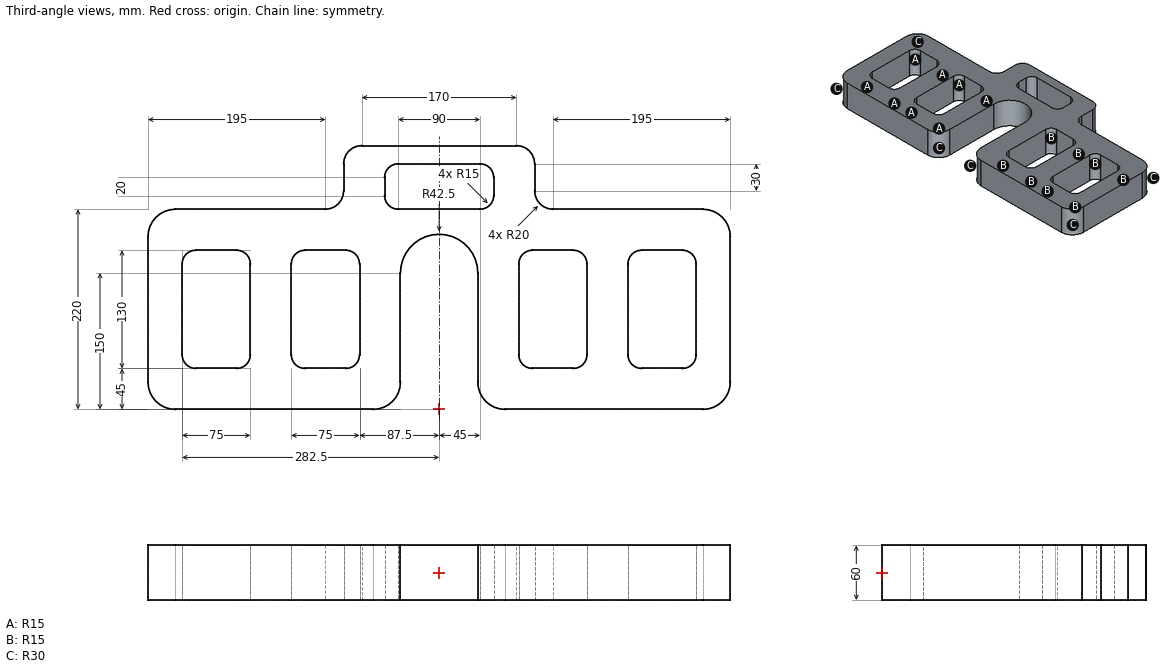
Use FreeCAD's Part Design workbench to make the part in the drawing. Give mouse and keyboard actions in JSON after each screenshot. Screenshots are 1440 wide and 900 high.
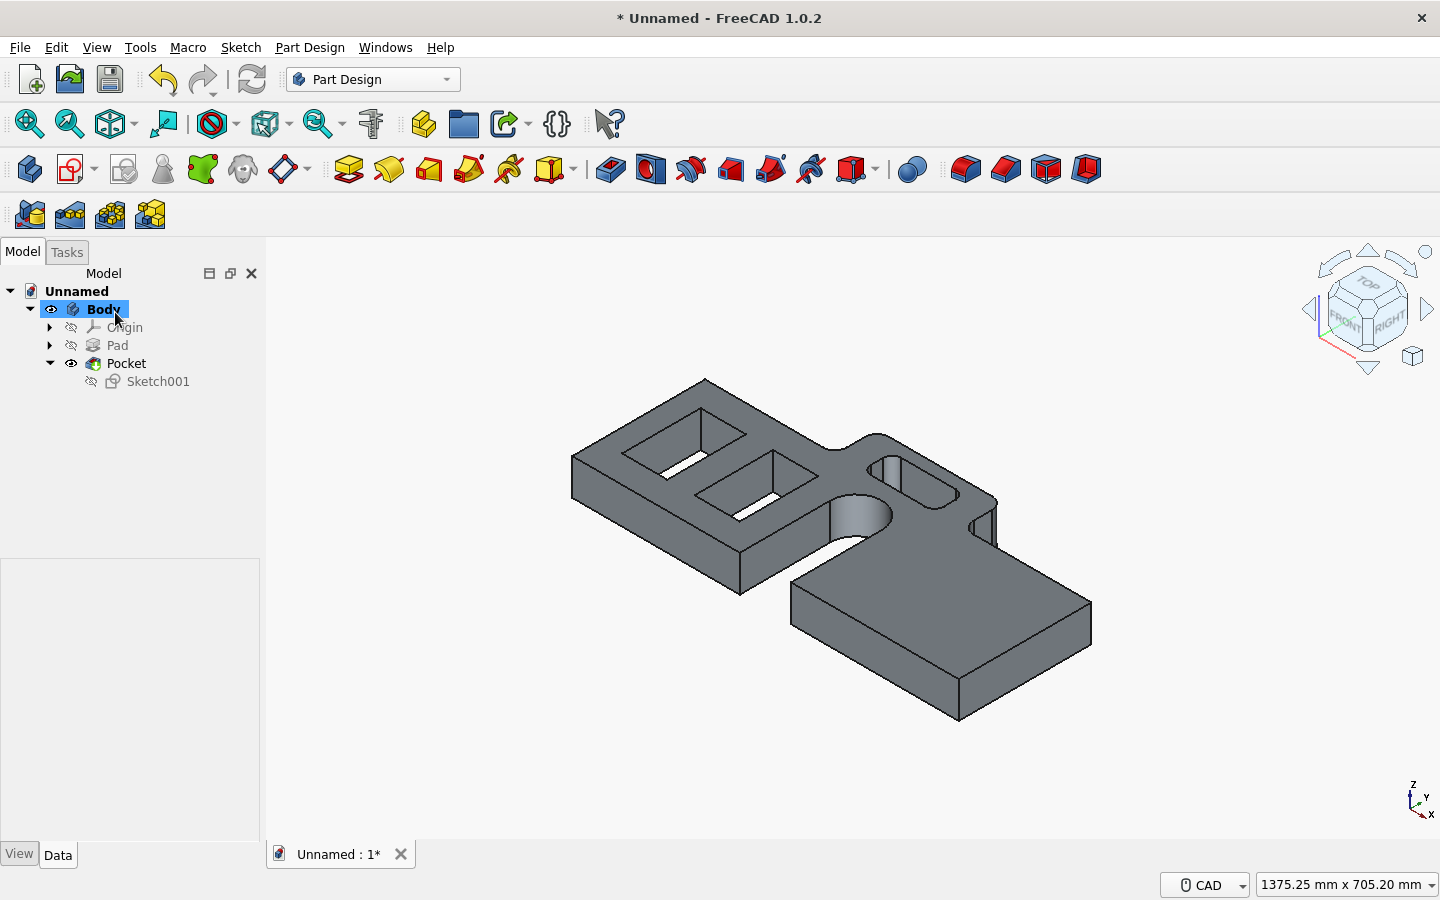
{"action": "key", "text": "2"}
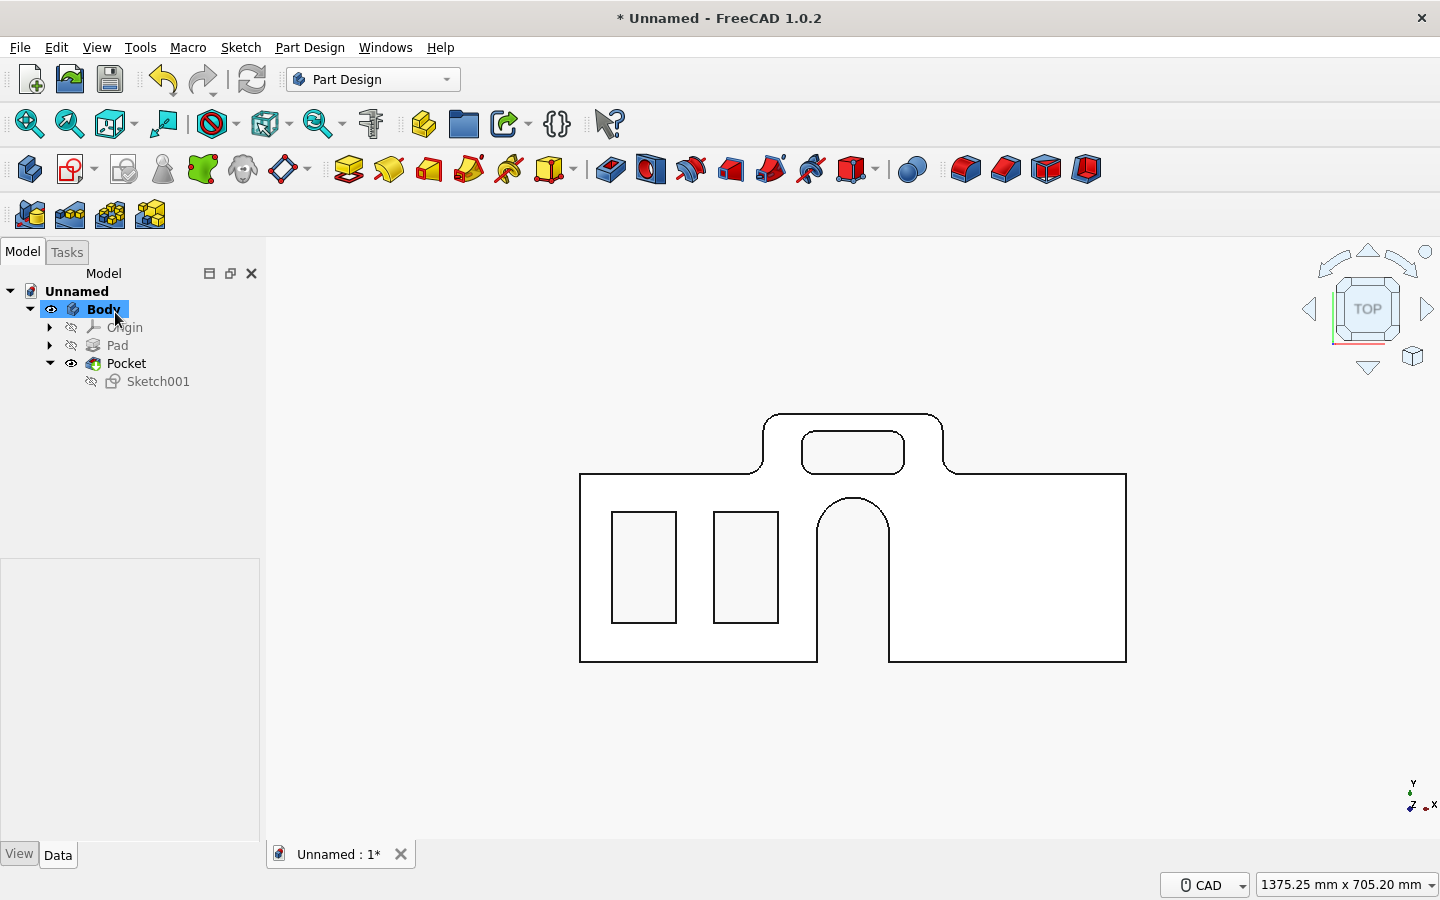
{"action": "key", "text": "1"}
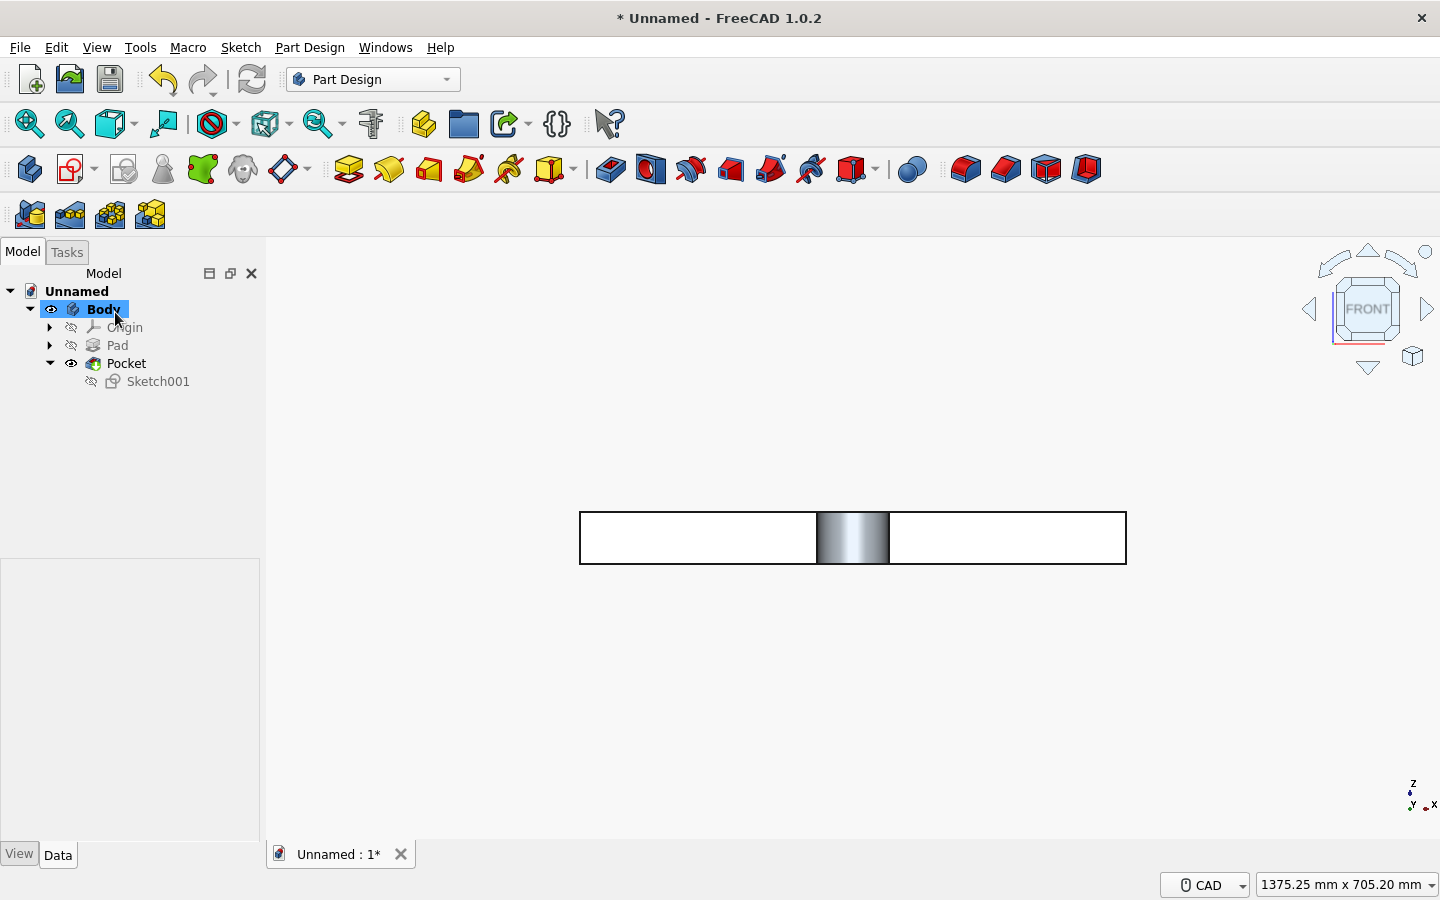
{"action": "key", "text": "3"}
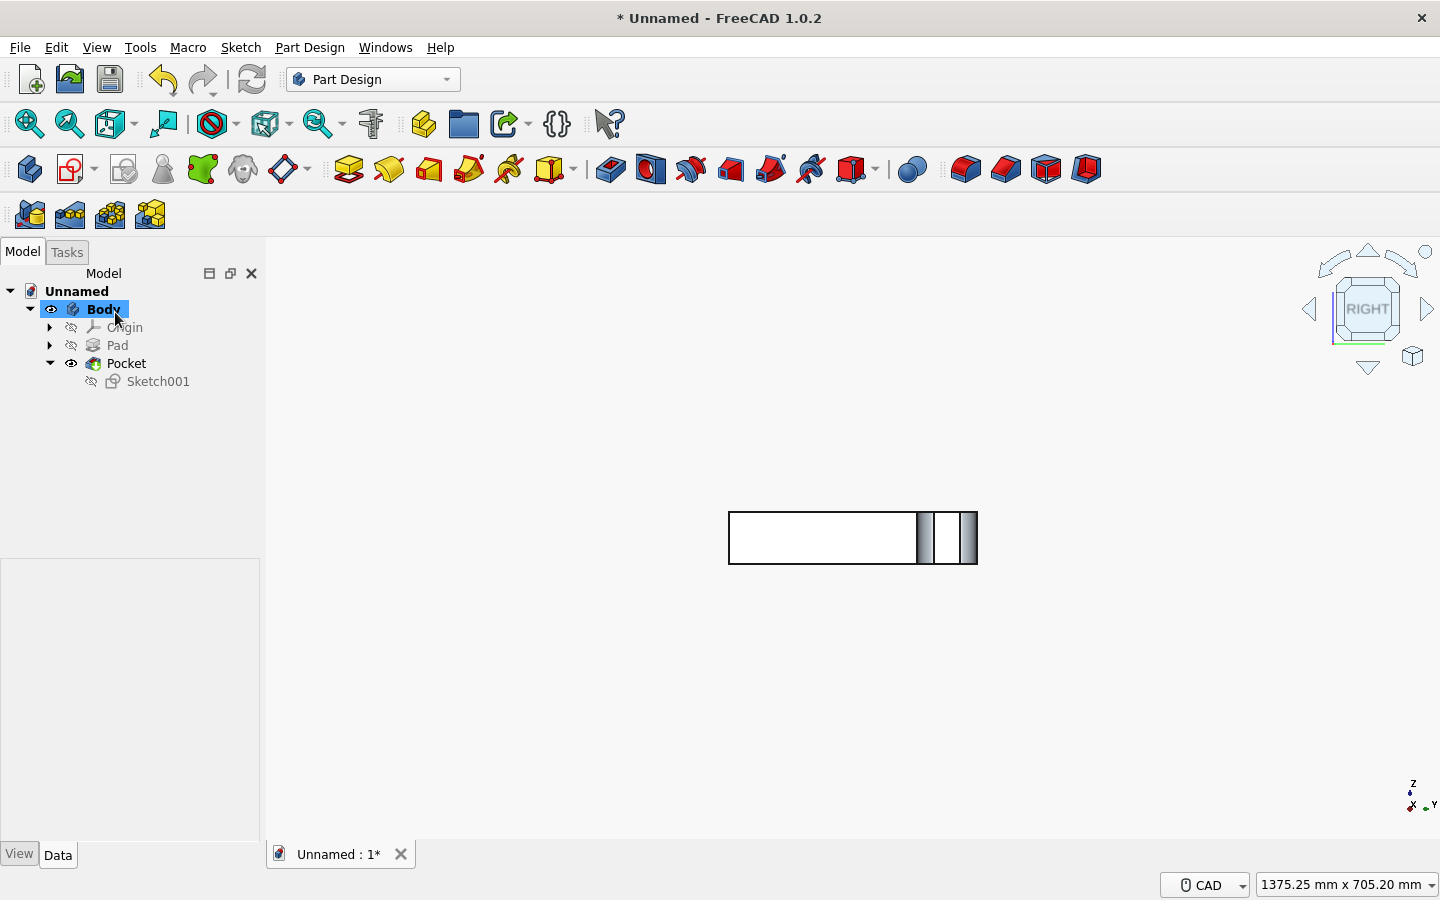
{"action": "key", "text": "v f"}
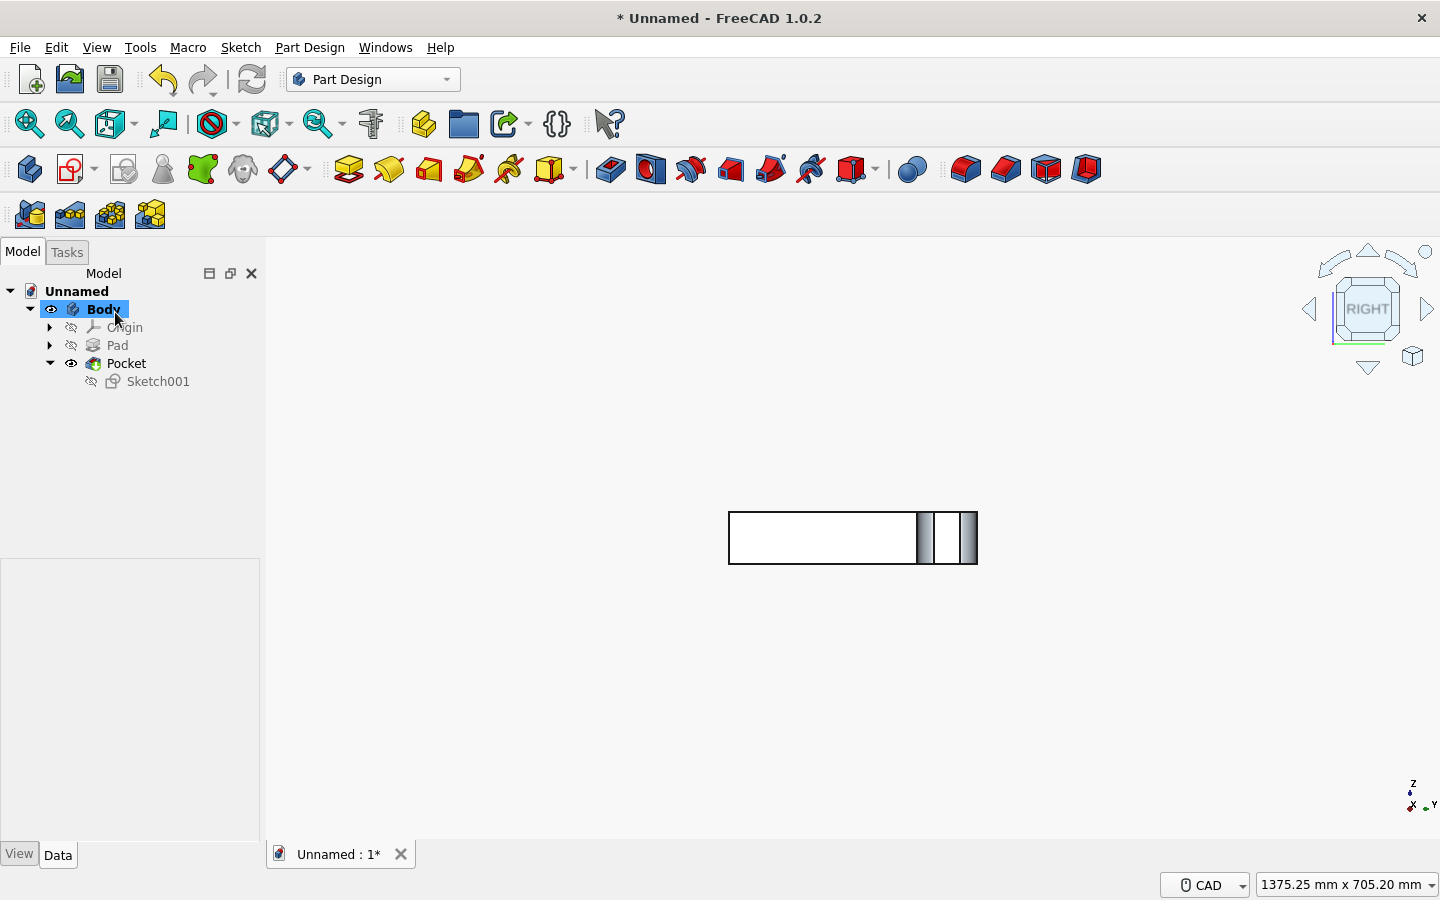
{"action": "key", "text": "5"}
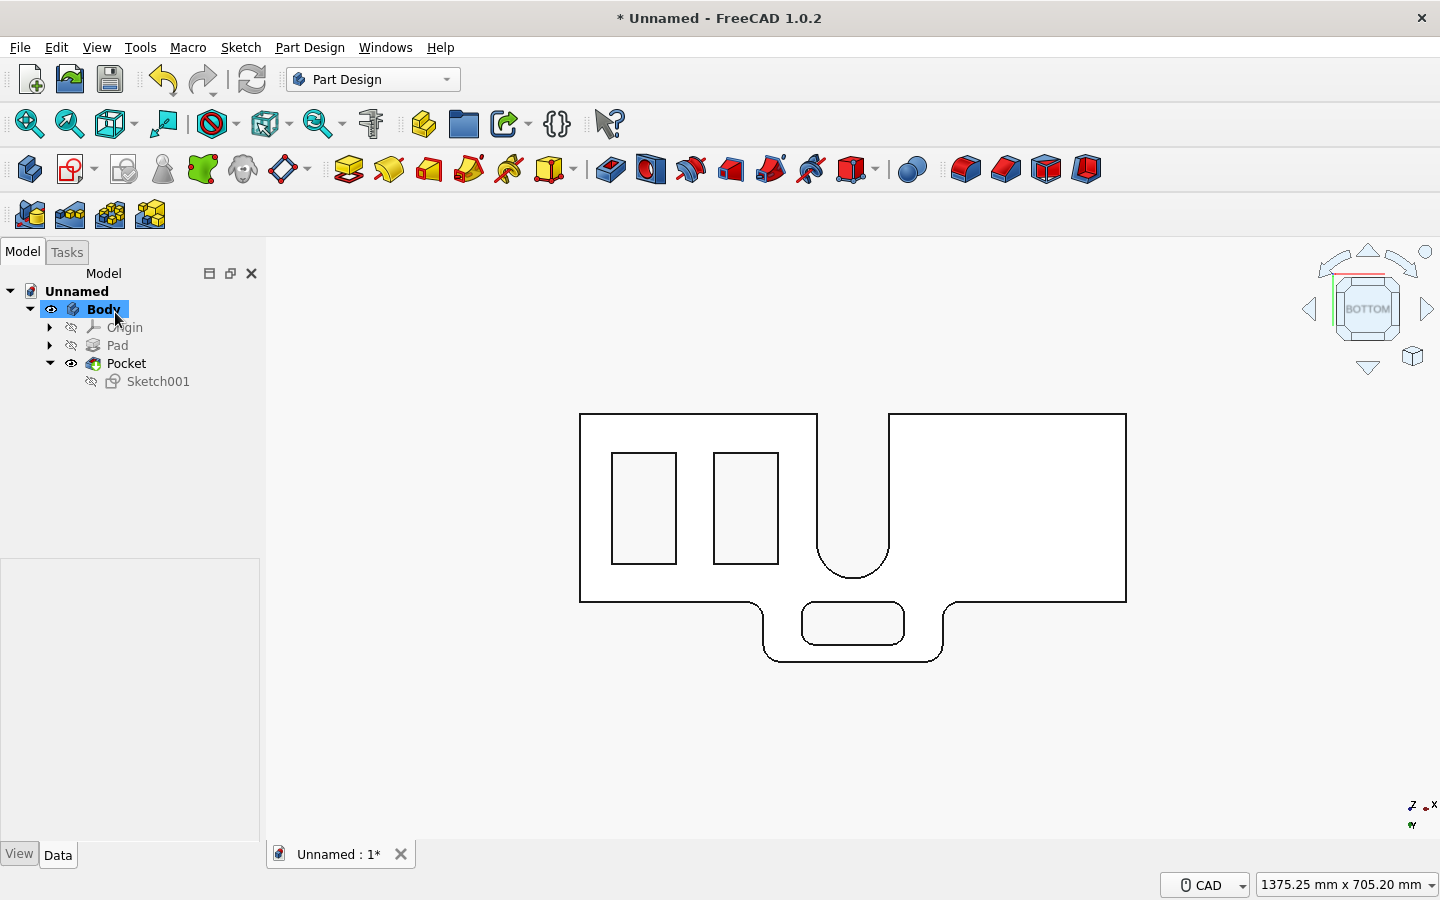
{"action": "key", "text": "4"}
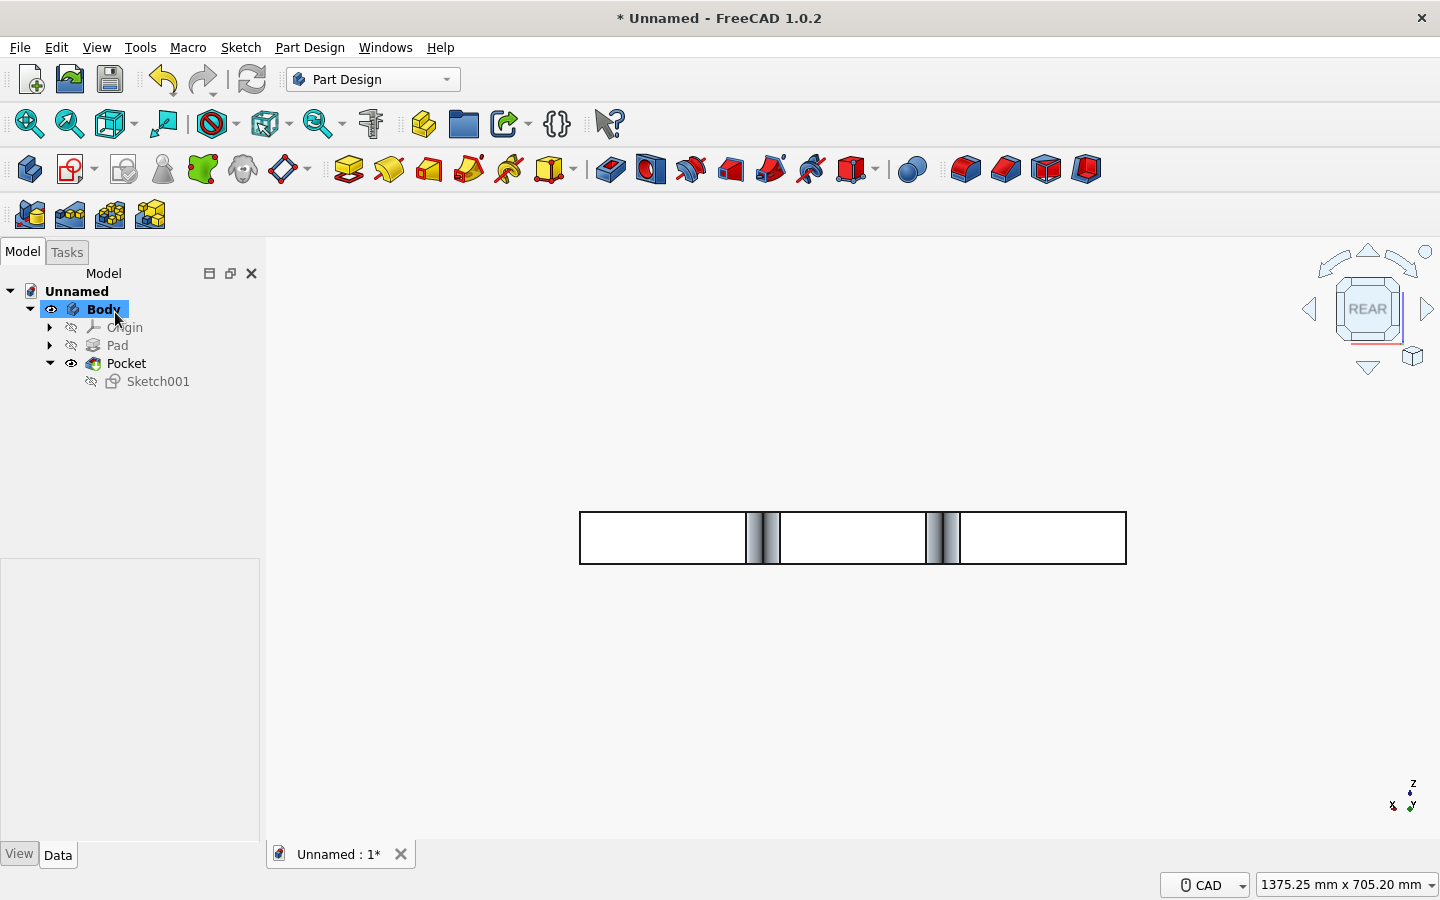
{"action": "key", "text": "6"}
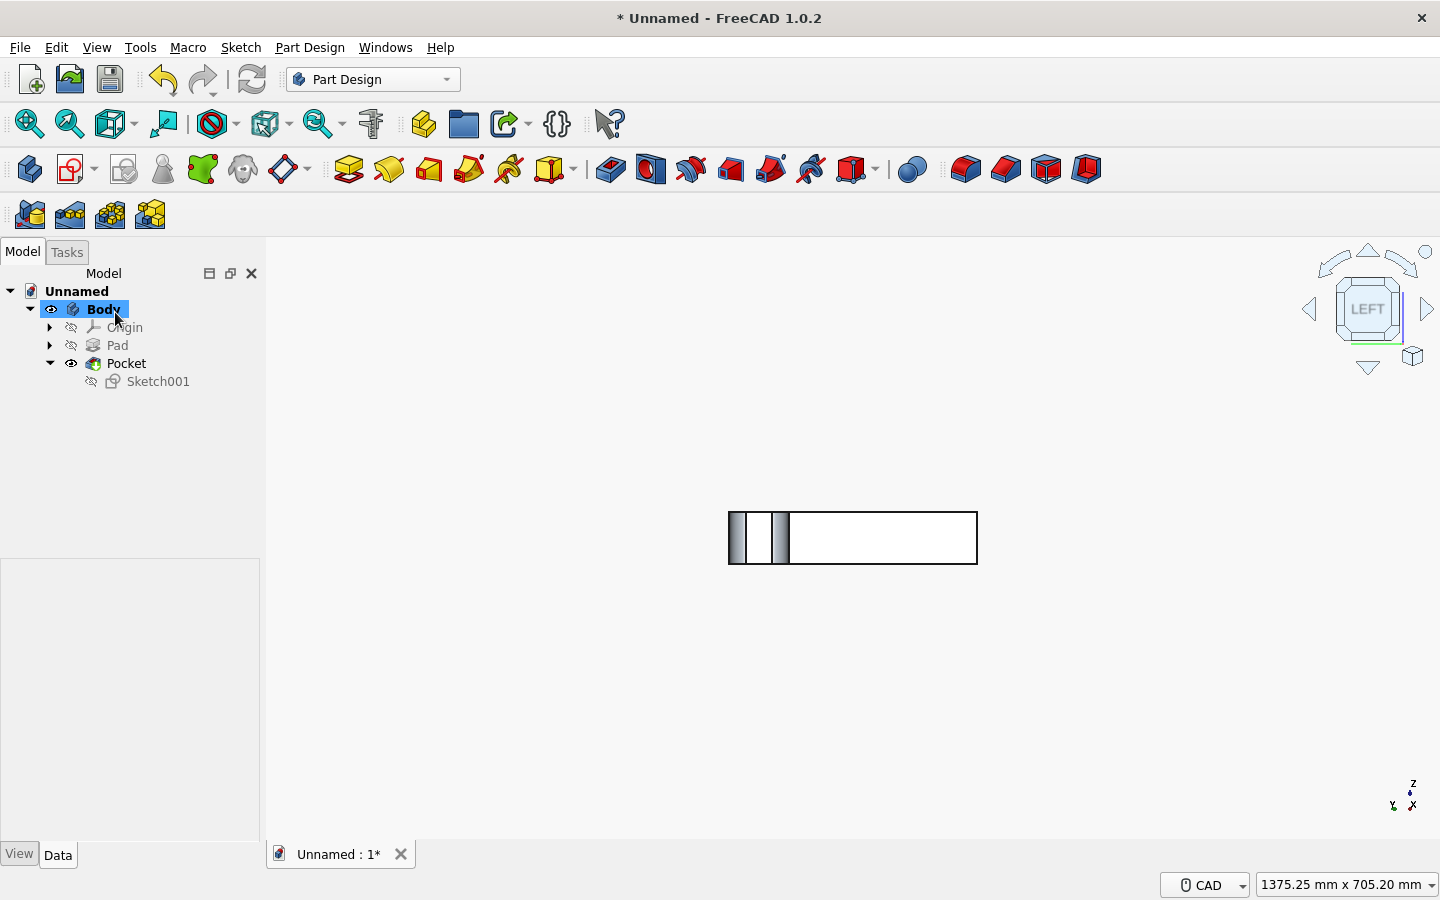
{"action": "left_click", "coordinate": [30, 124]}